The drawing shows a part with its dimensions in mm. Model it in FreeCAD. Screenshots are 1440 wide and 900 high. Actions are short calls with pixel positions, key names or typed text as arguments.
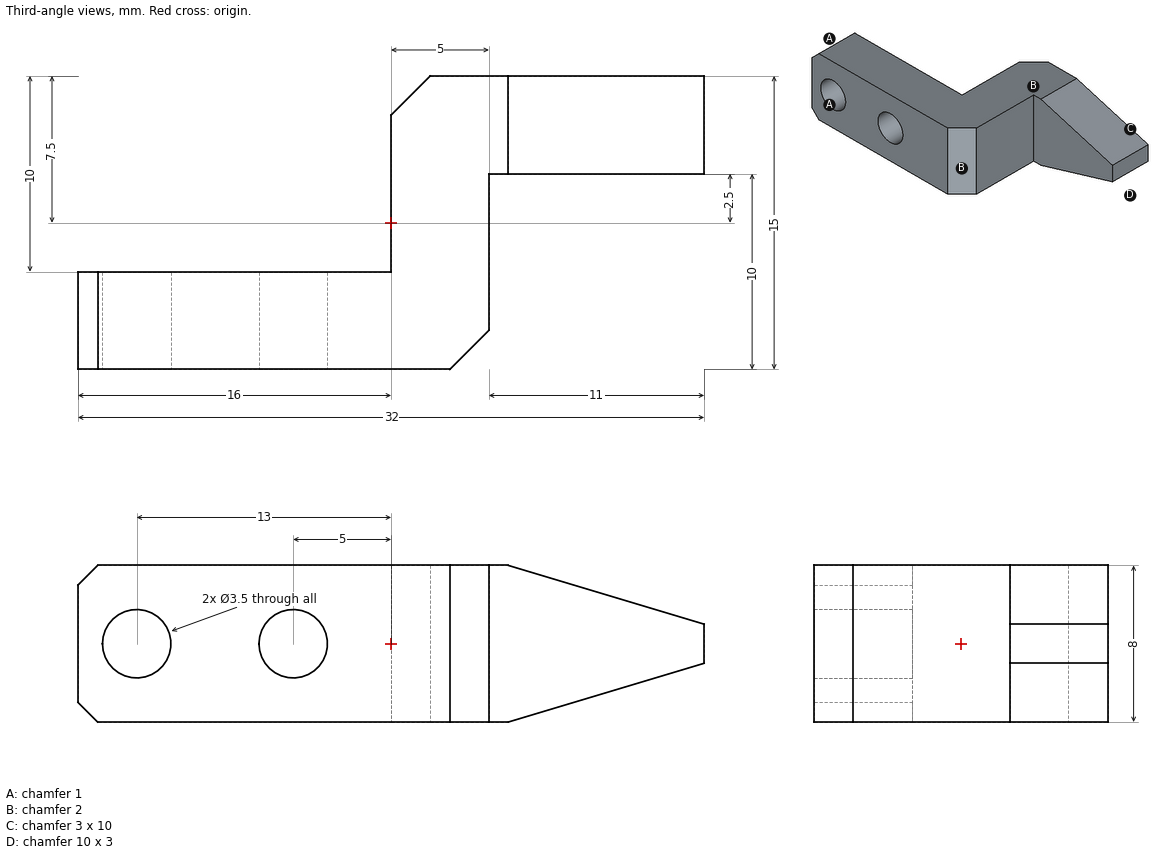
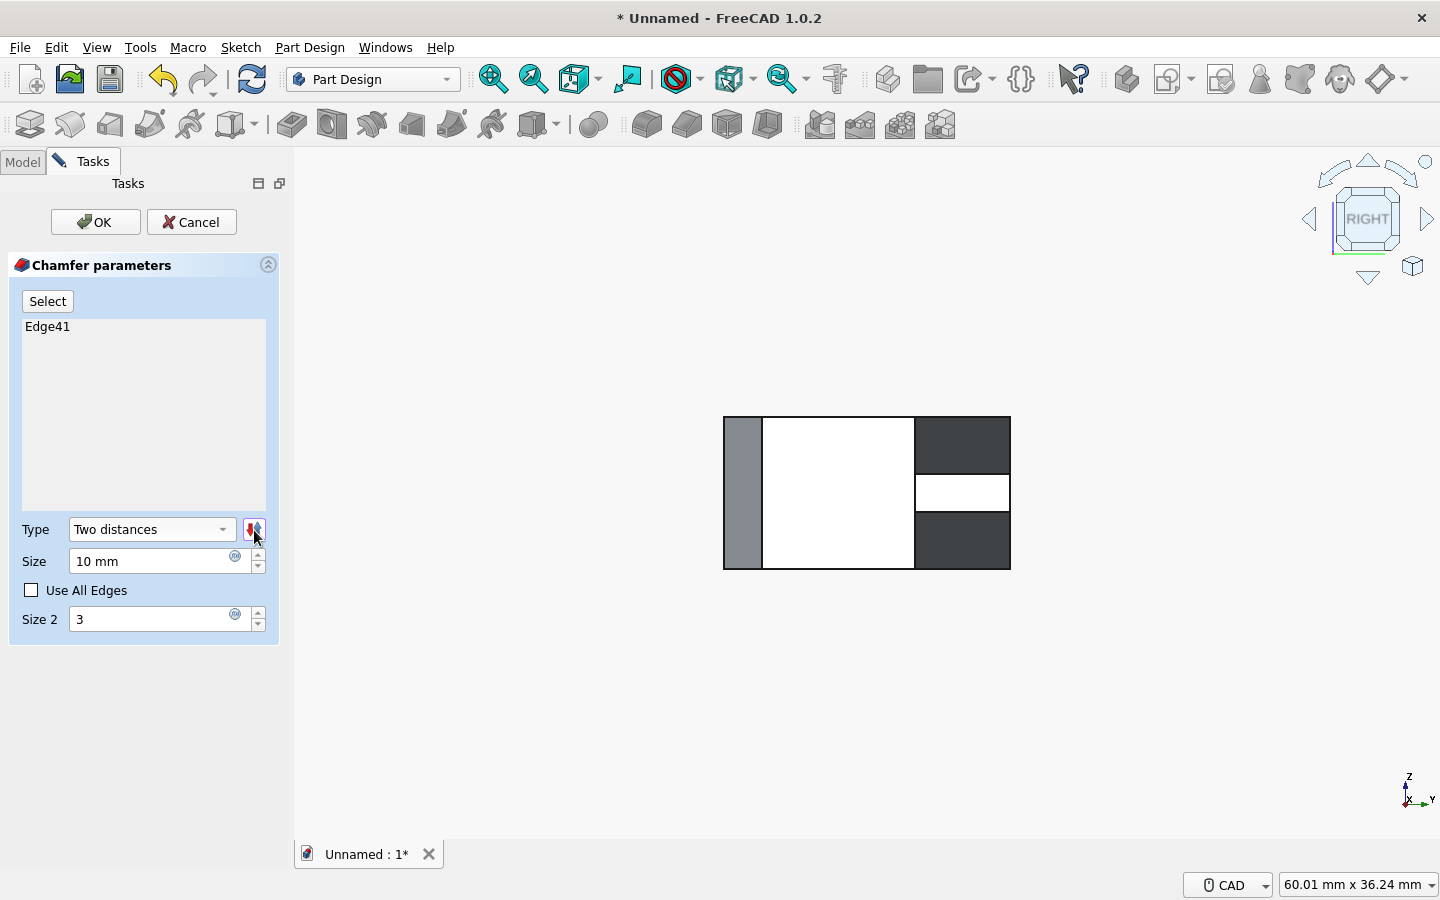
click(96, 222)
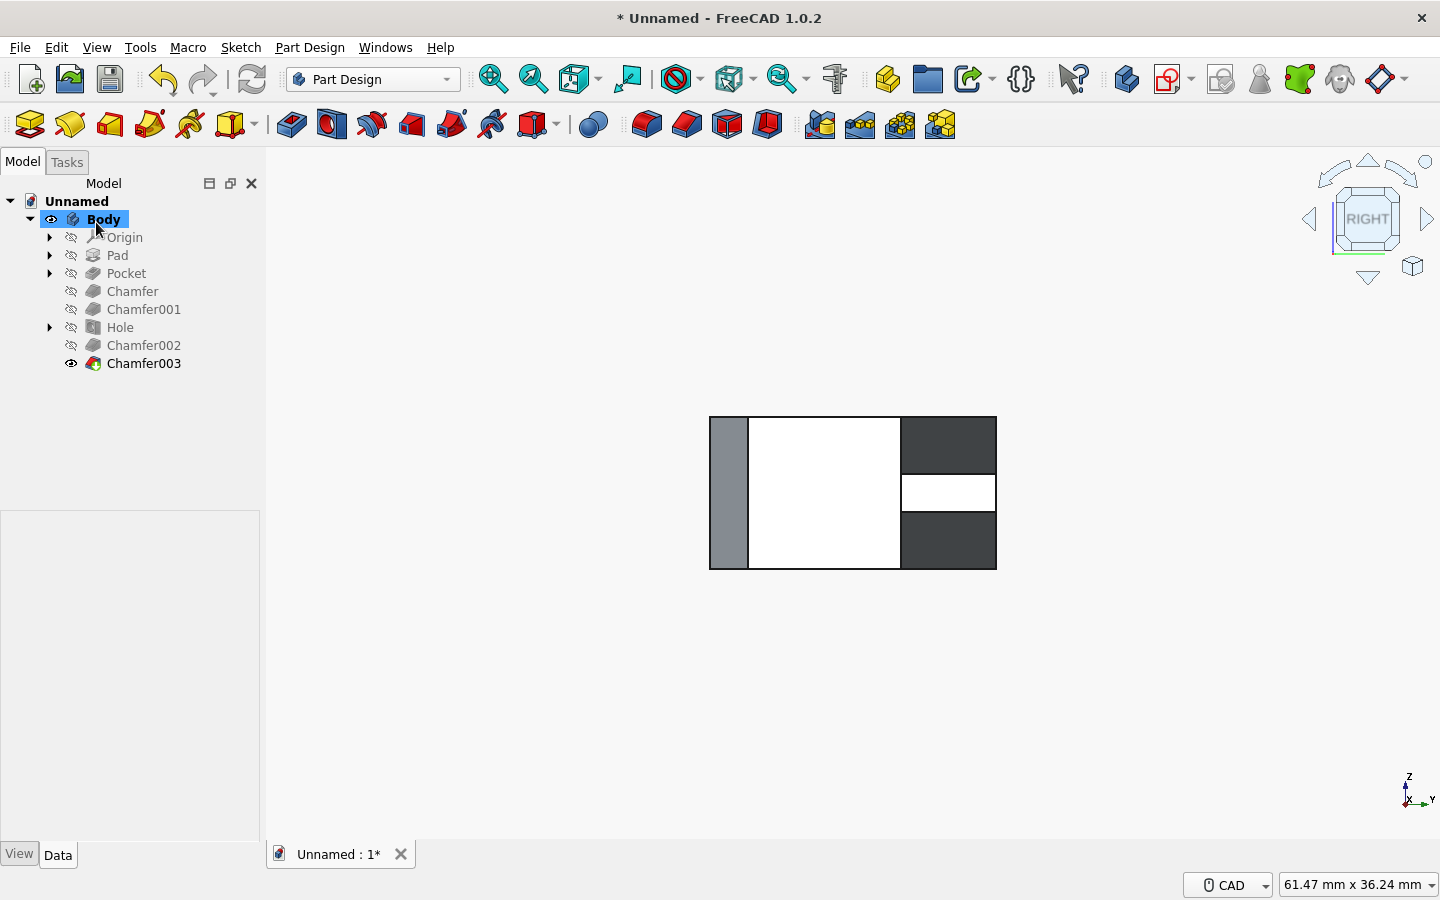
key(0)